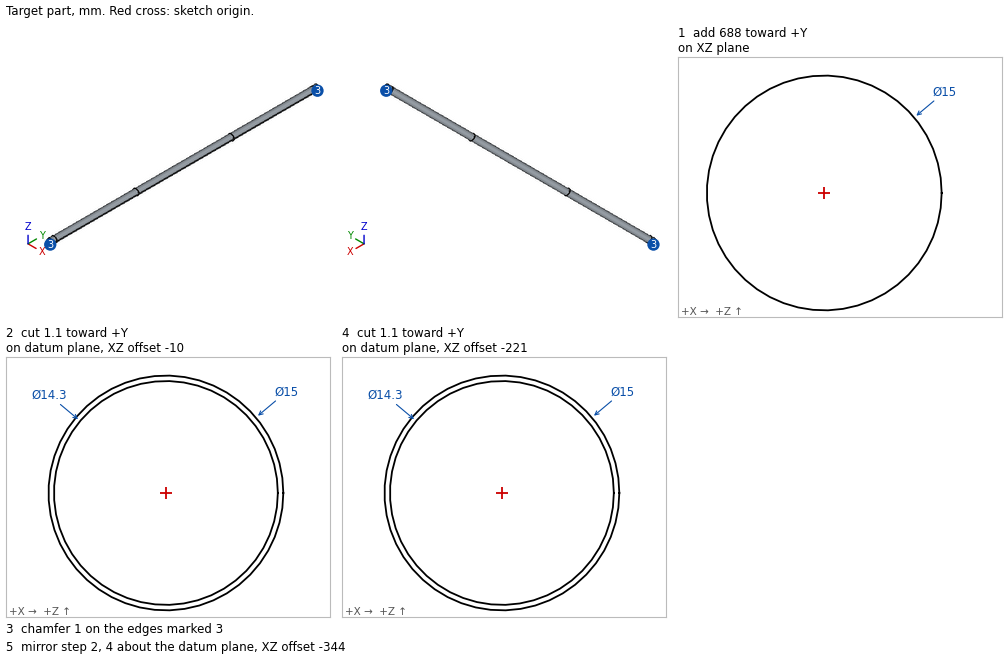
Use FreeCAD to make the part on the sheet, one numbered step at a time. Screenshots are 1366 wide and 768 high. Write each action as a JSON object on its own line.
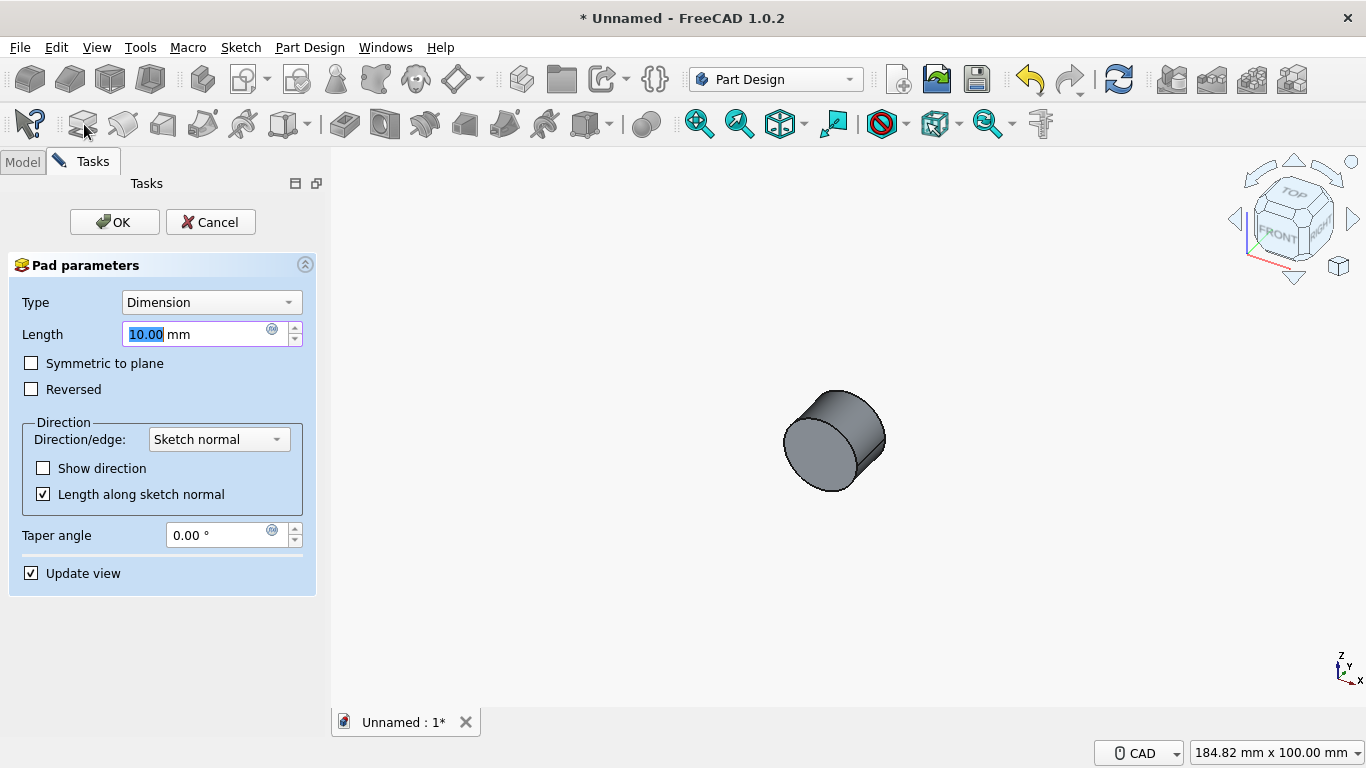
{"action": "type", "text": "688"}
{"action": "key", "text": "Tab"}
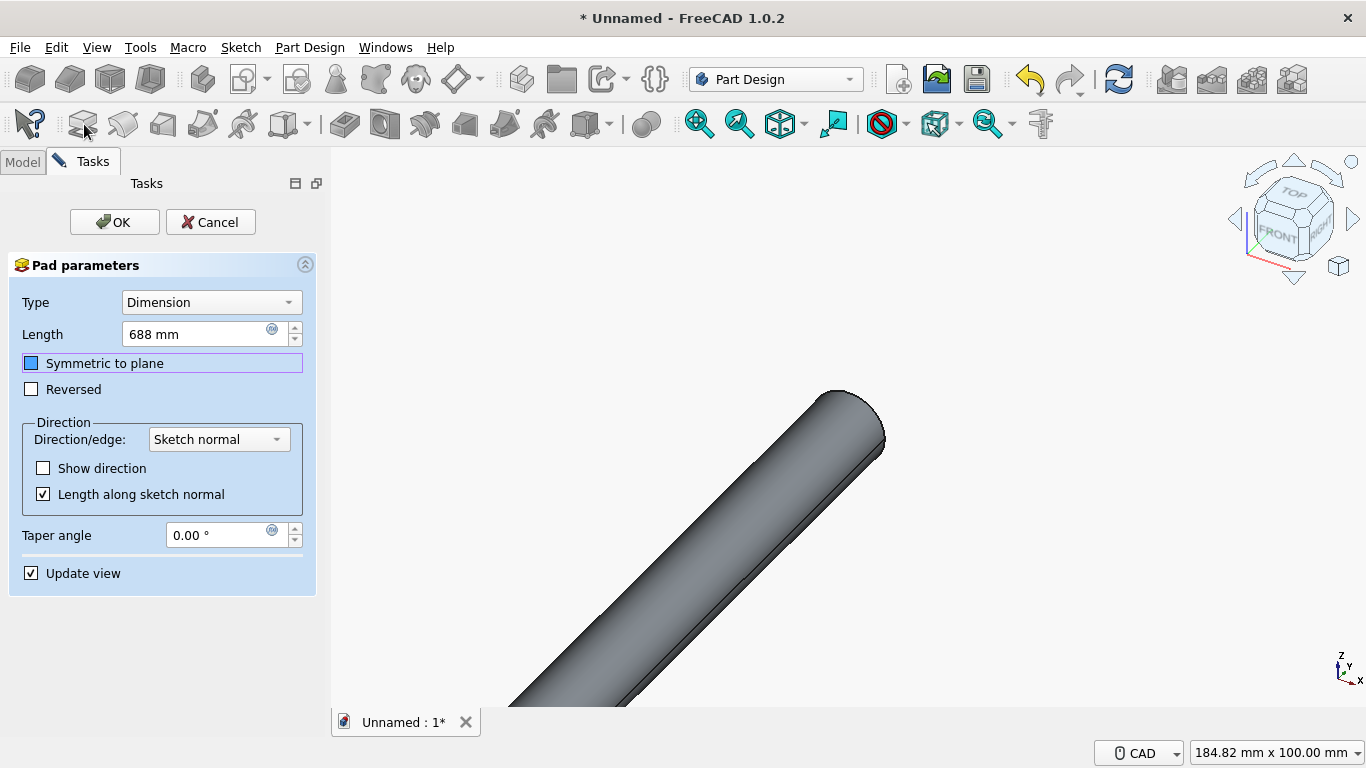
{"action": "left_click", "coordinate": [30, 389]}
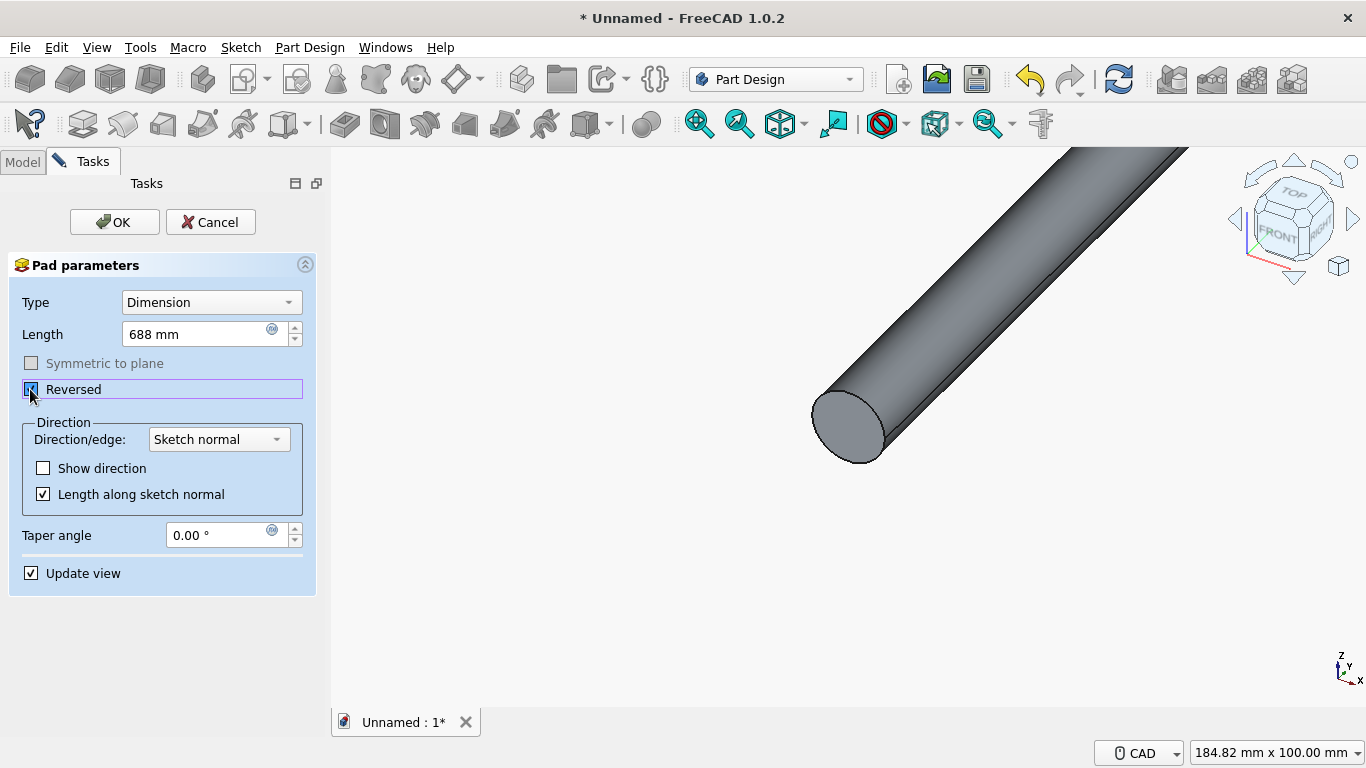
{"action": "left_click", "coordinate": [115, 222]}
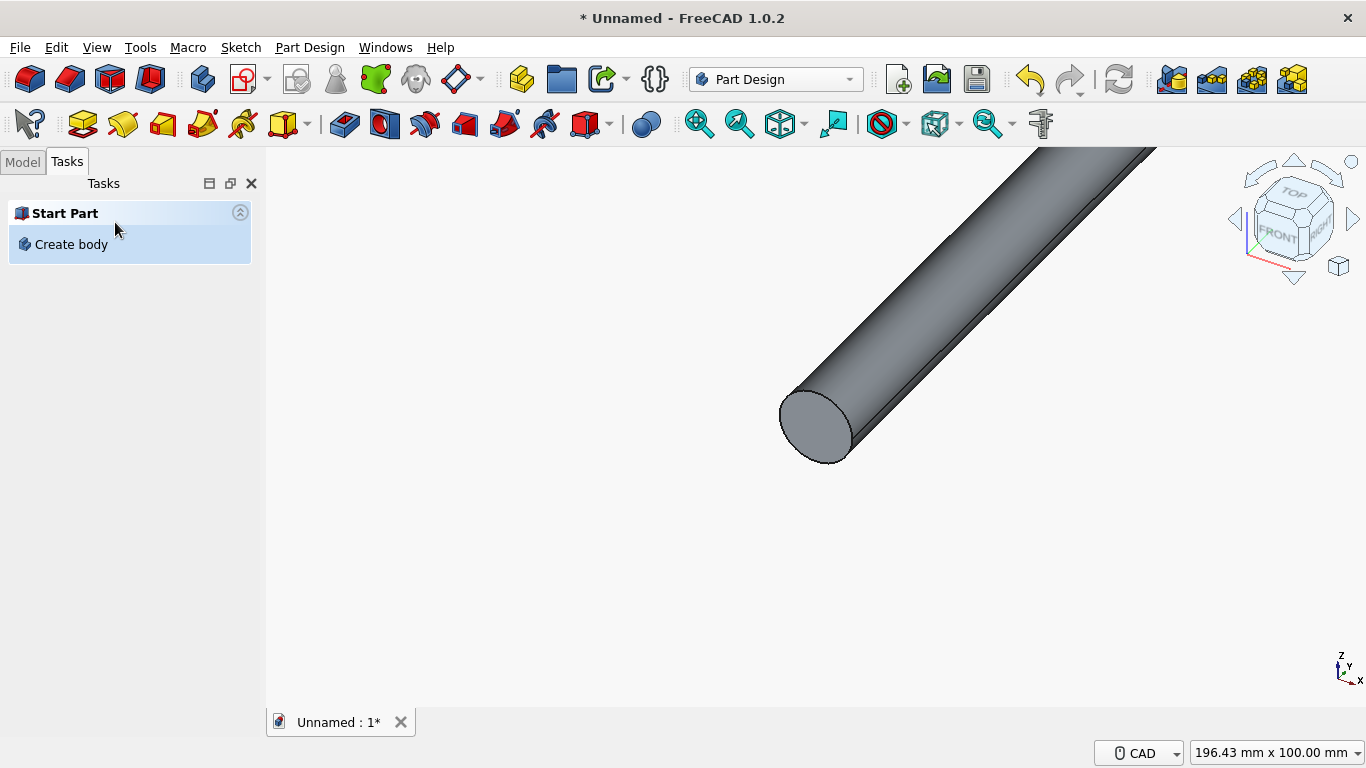
{"action": "left_click", "coordinate": [700, 124]}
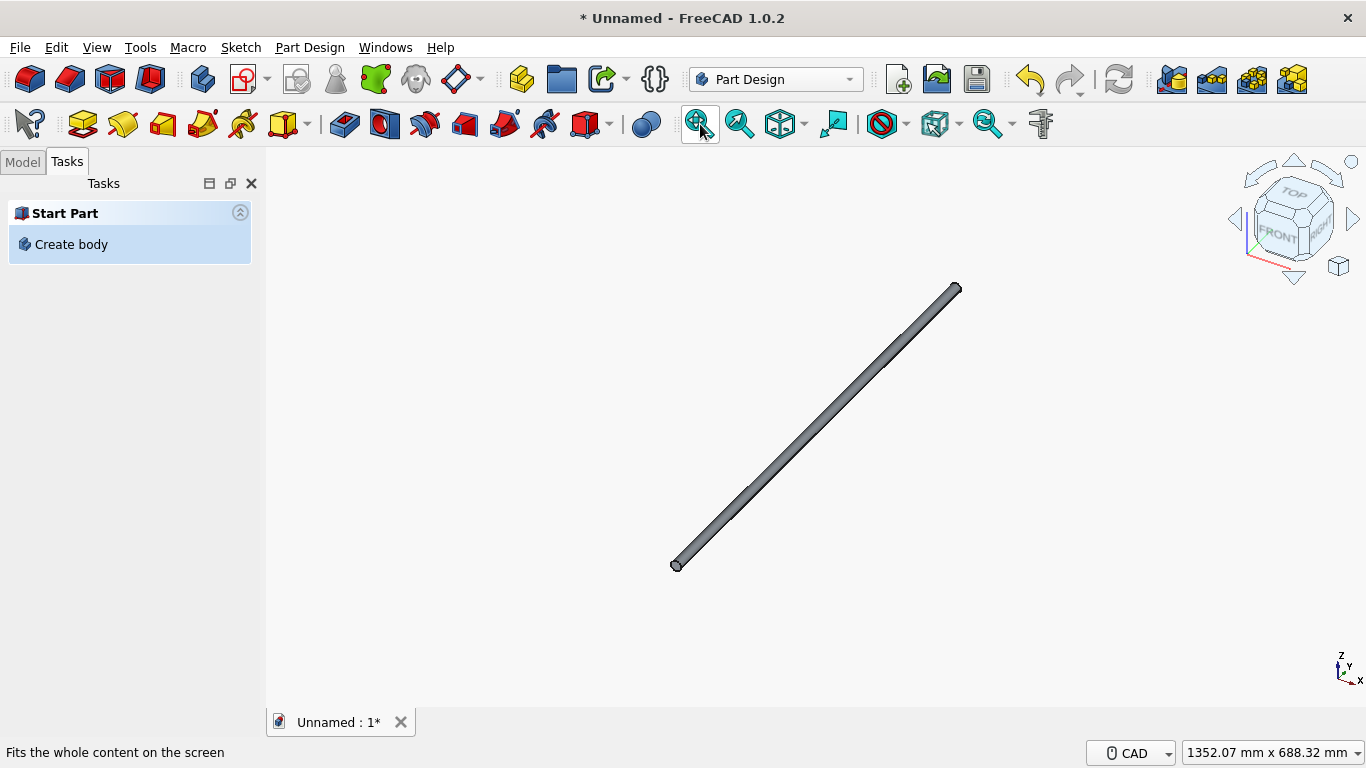
{"action": "left_click", "coordinate": [23, 161]}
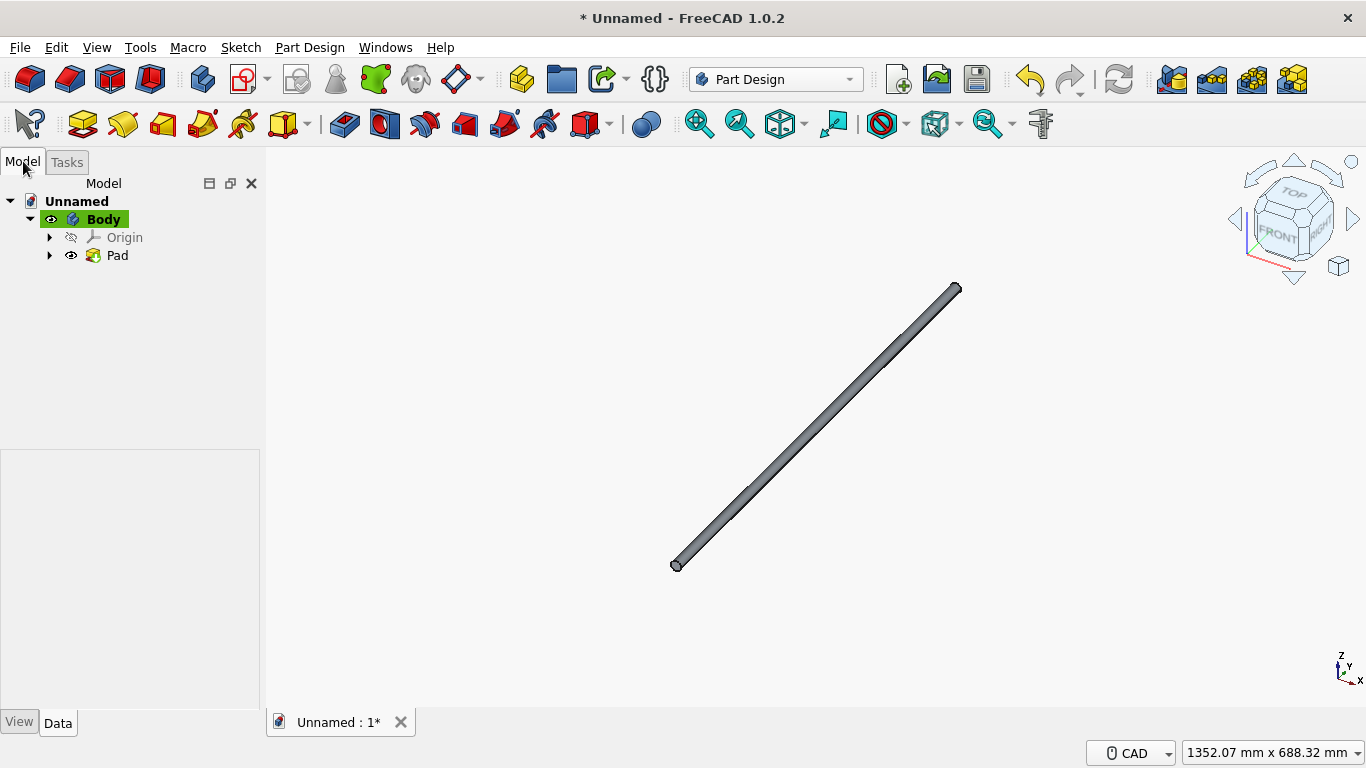
{"action": "left_click", "coordinate": [50, 237]}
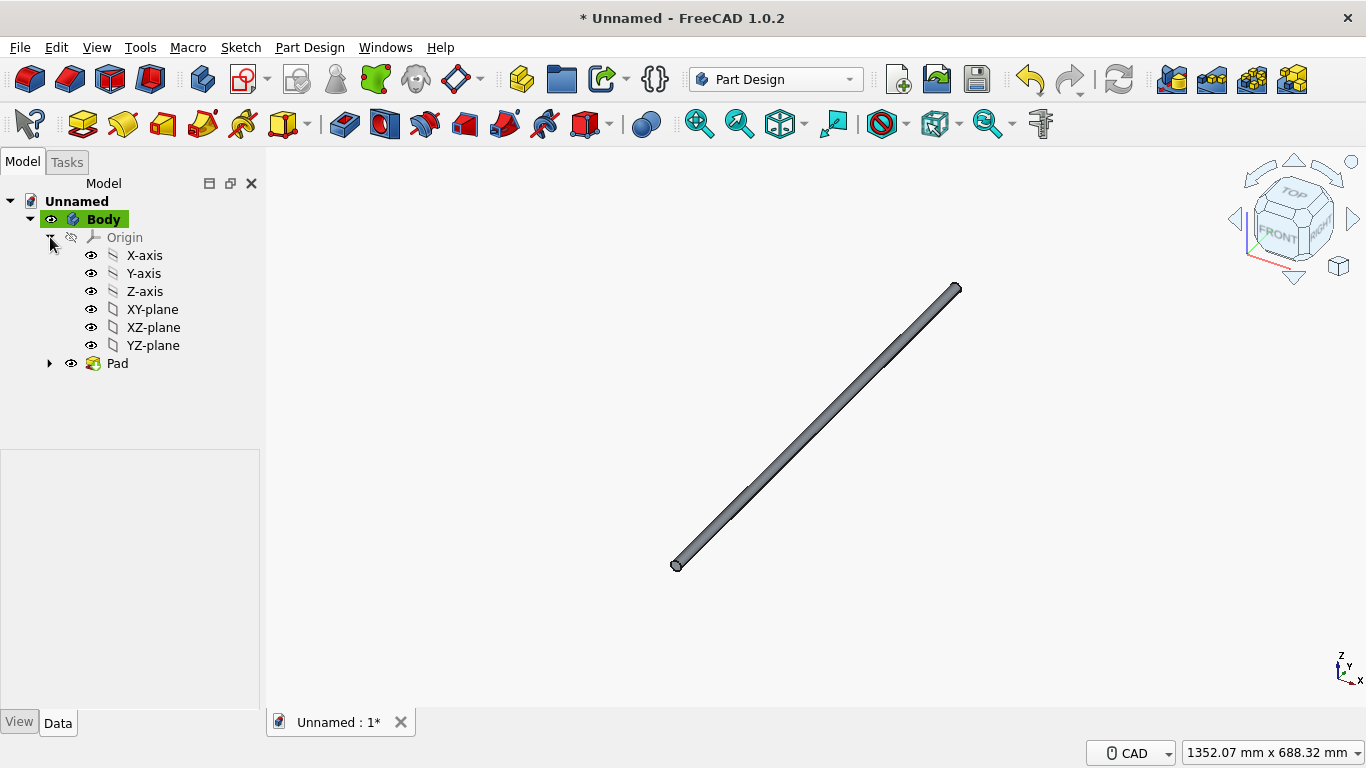
{"action": "left_click", "coordinate": [136, 327]}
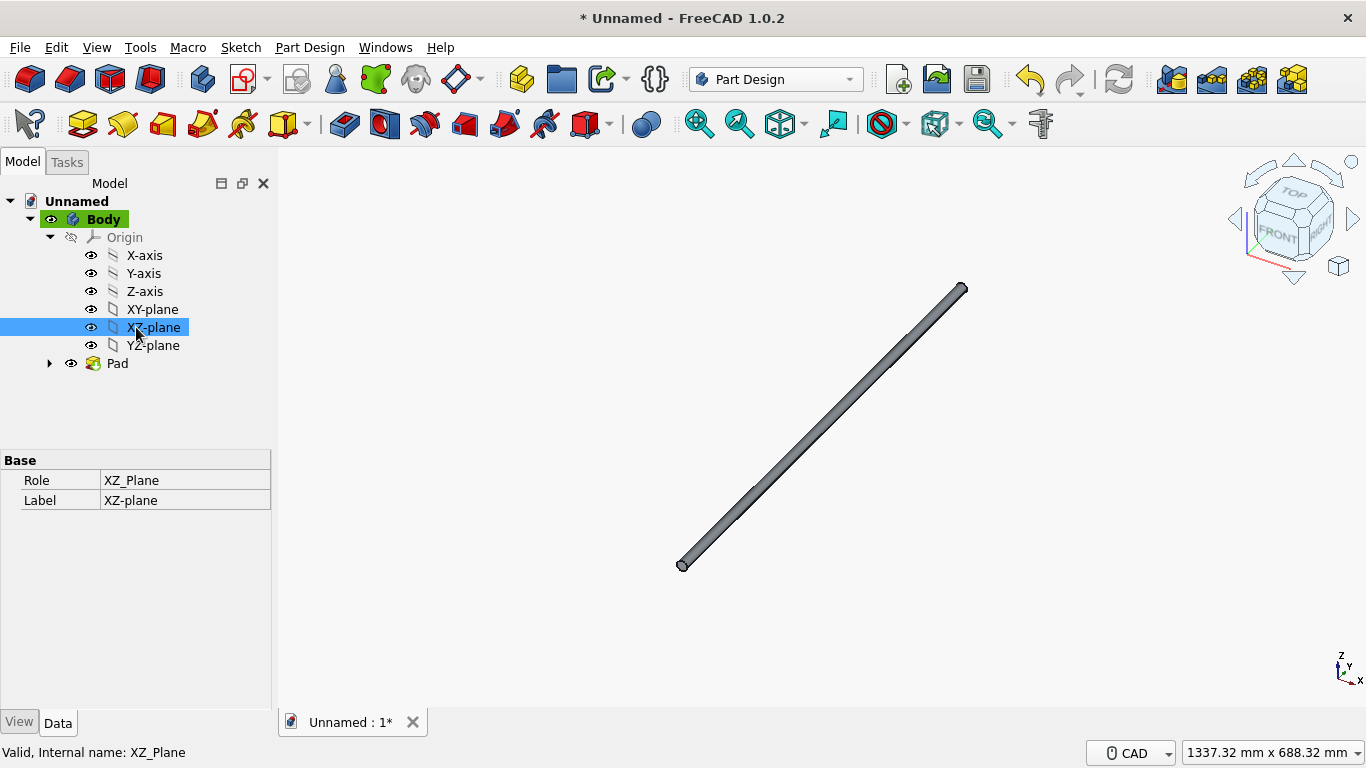
{"action": "left_click", "coordinate": [456, 80]}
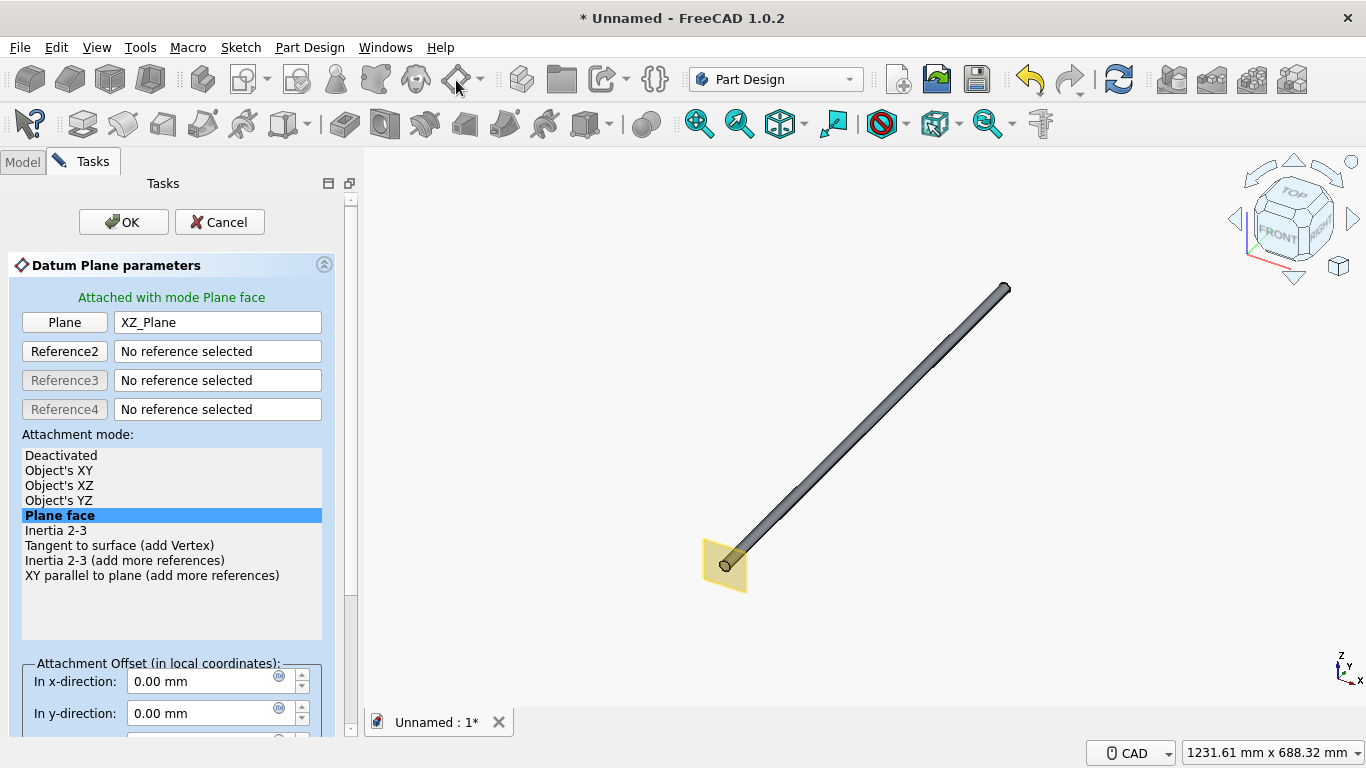
{"action": "scroll", "coordinate": [351, 464], "scroll_direction": "down", "scroll_amount": 2}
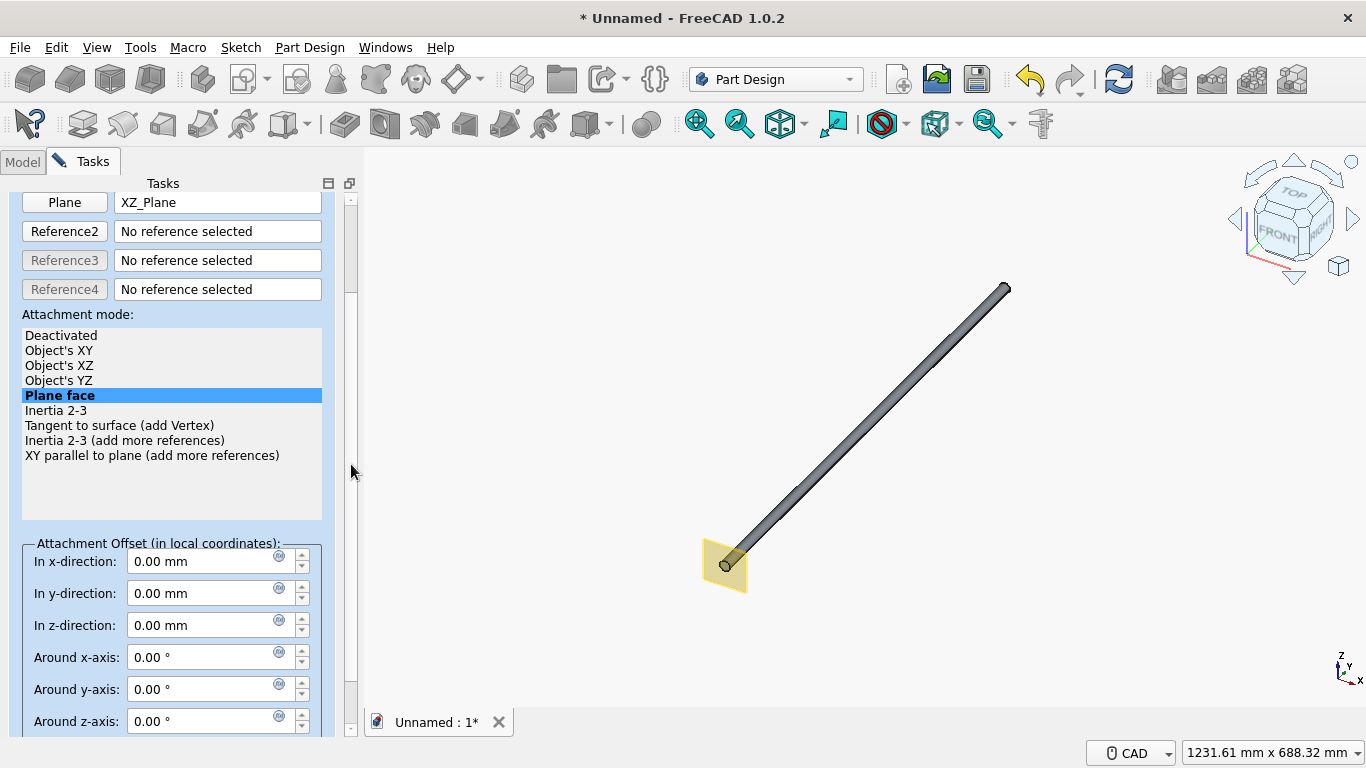
{"action": "triple_click", "coordinate": [210, 625]}